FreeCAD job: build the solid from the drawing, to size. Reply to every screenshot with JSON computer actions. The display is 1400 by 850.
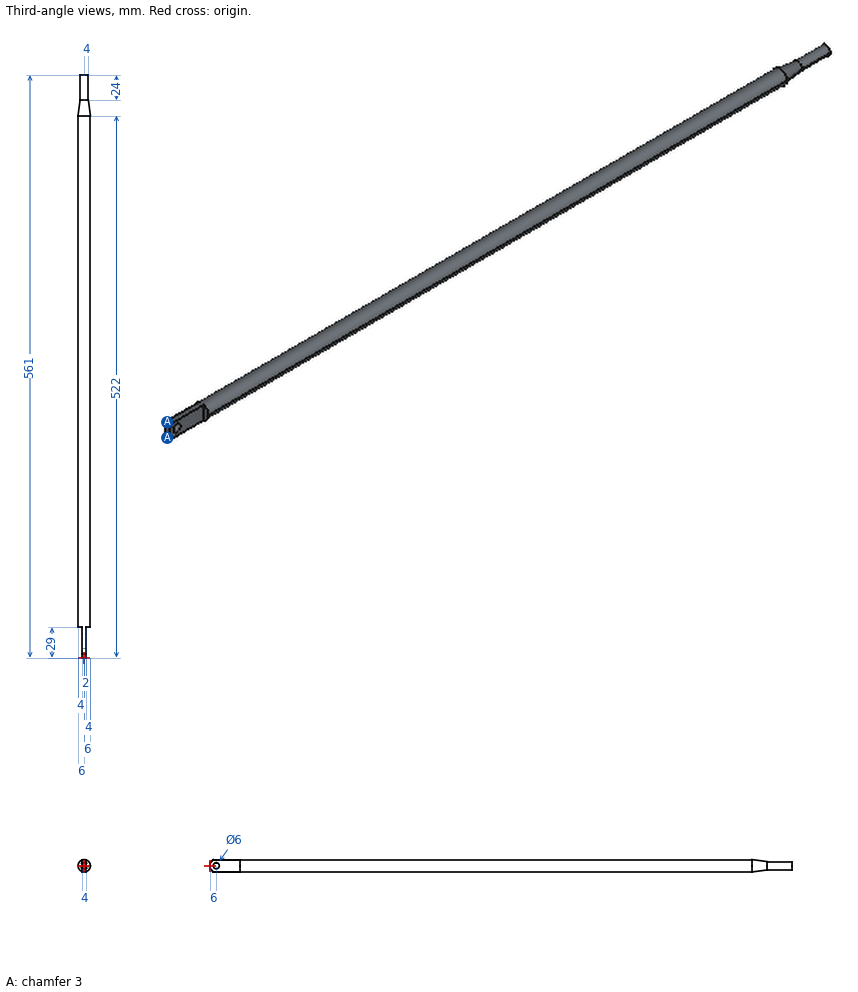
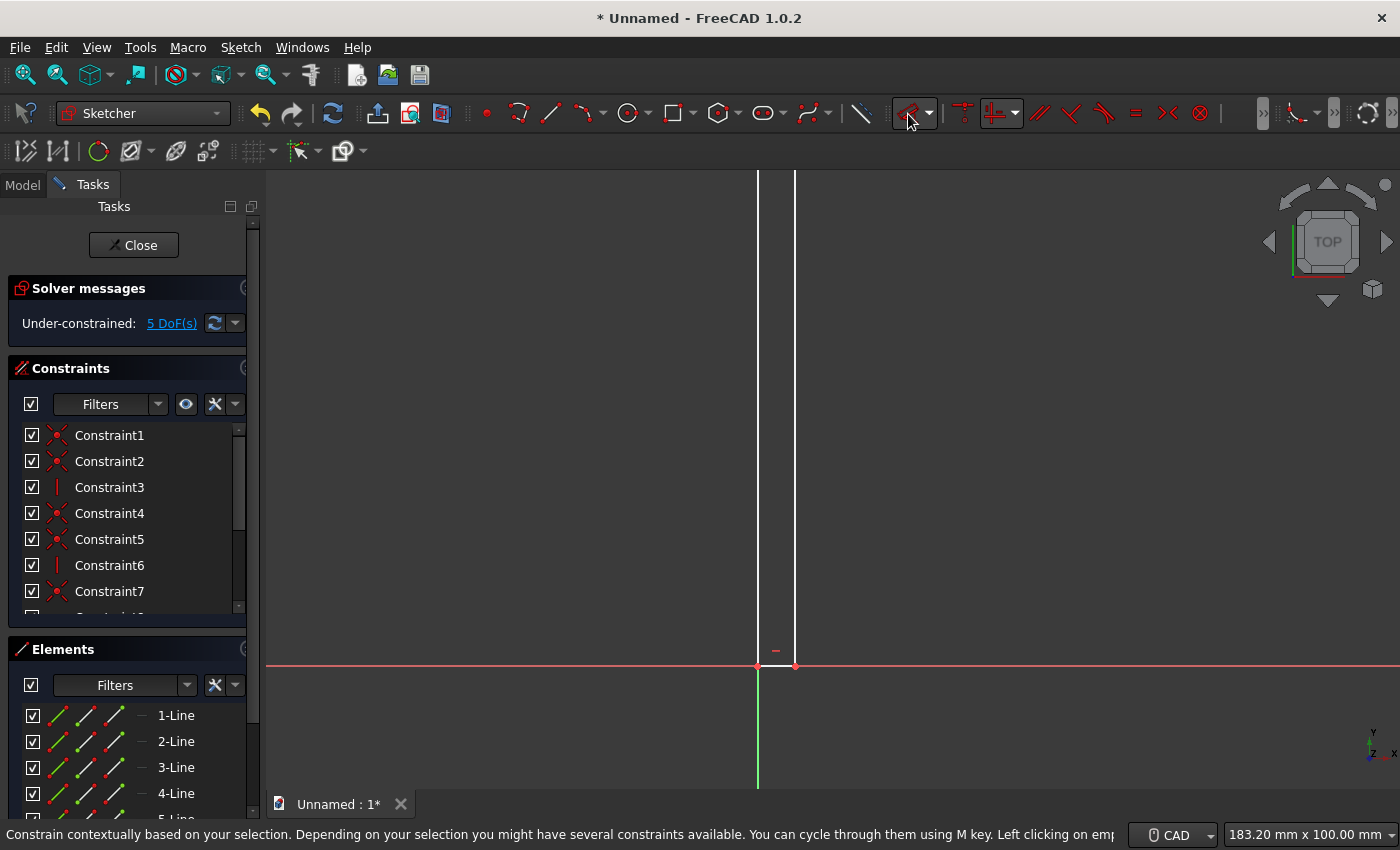
{"action": "left_click", "coordinate": [769, 666]}
{"action": "left_click", "coordinate": [777, 700]}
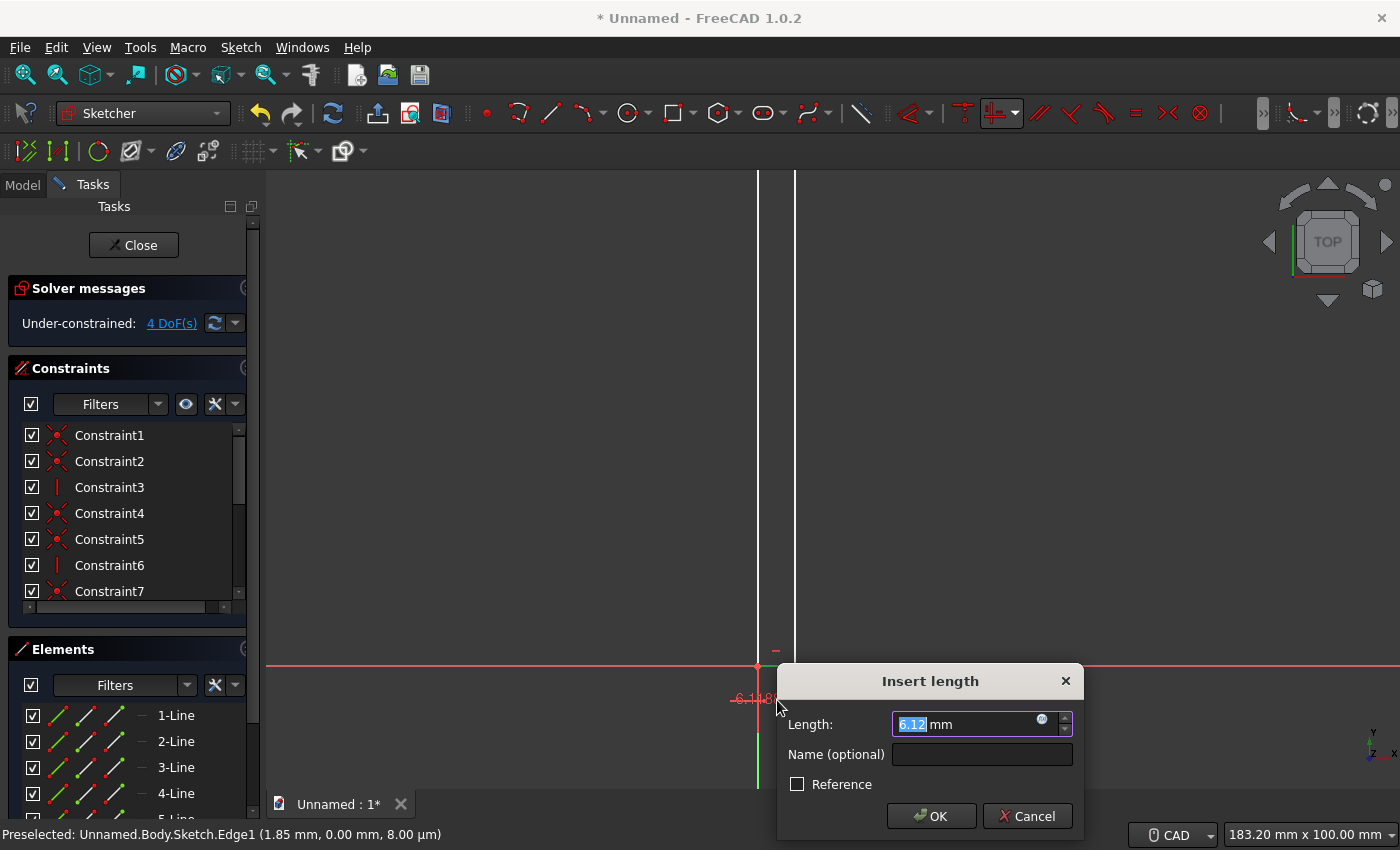
{"action": "type", "text": "6"}
{"action": "key", "text": "Return"}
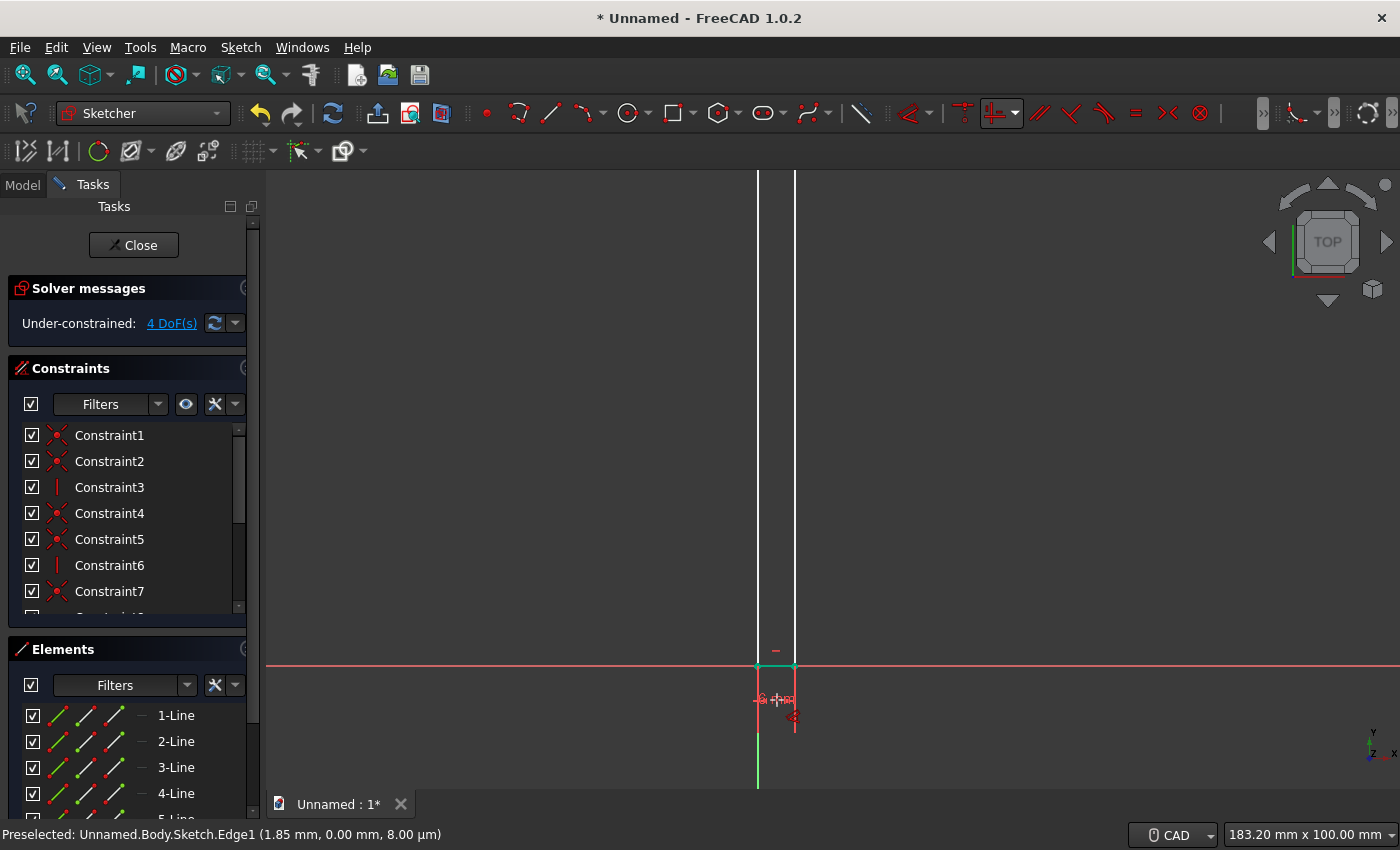
{"action": "scroll", "coordinate": [763, 673], "scroll_direction": "down", "scroll_amount": 11}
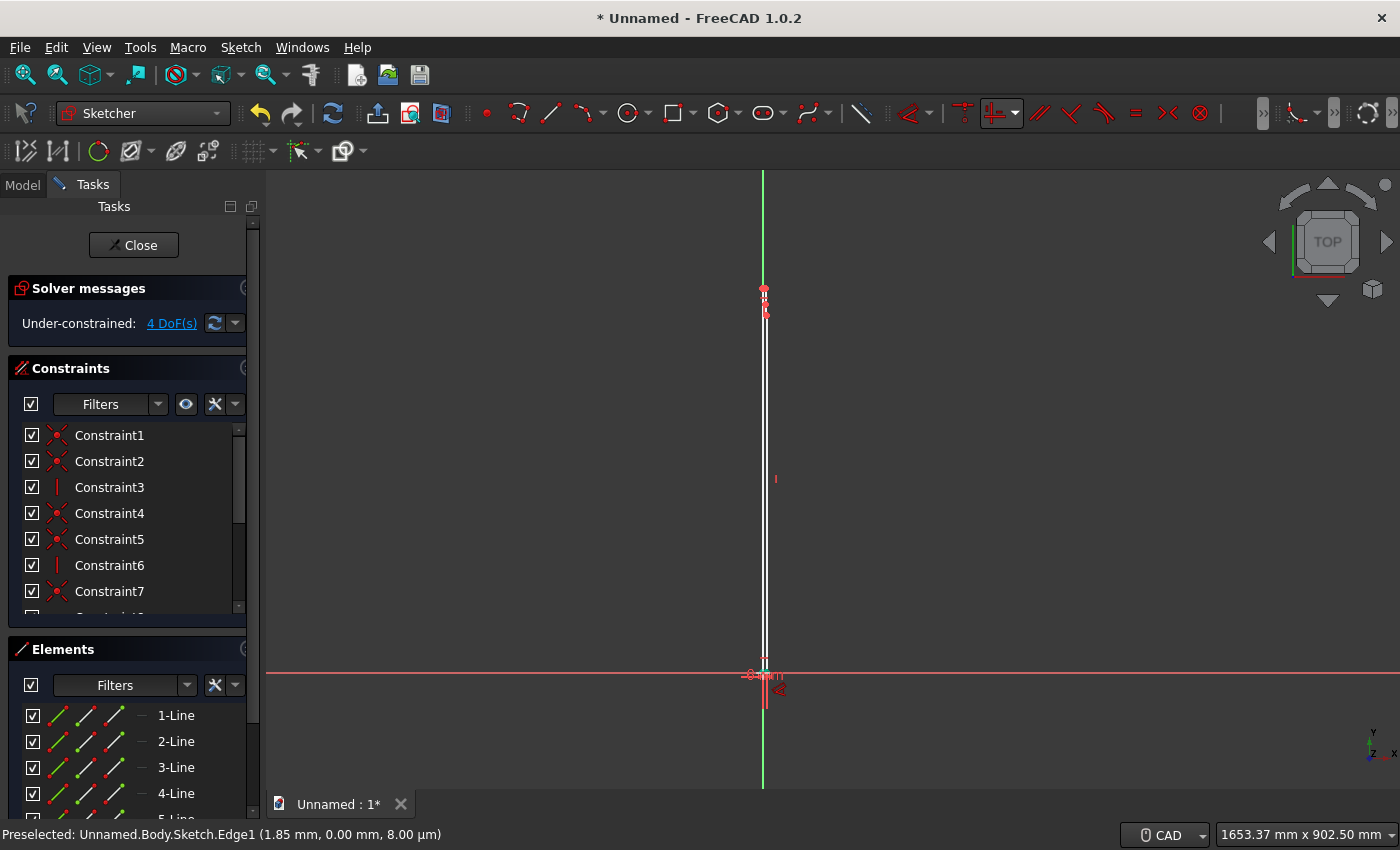
{"action": "scroll", "coordinate": [764, 288], "scroll_direction": "up", "scroll_amount": 14}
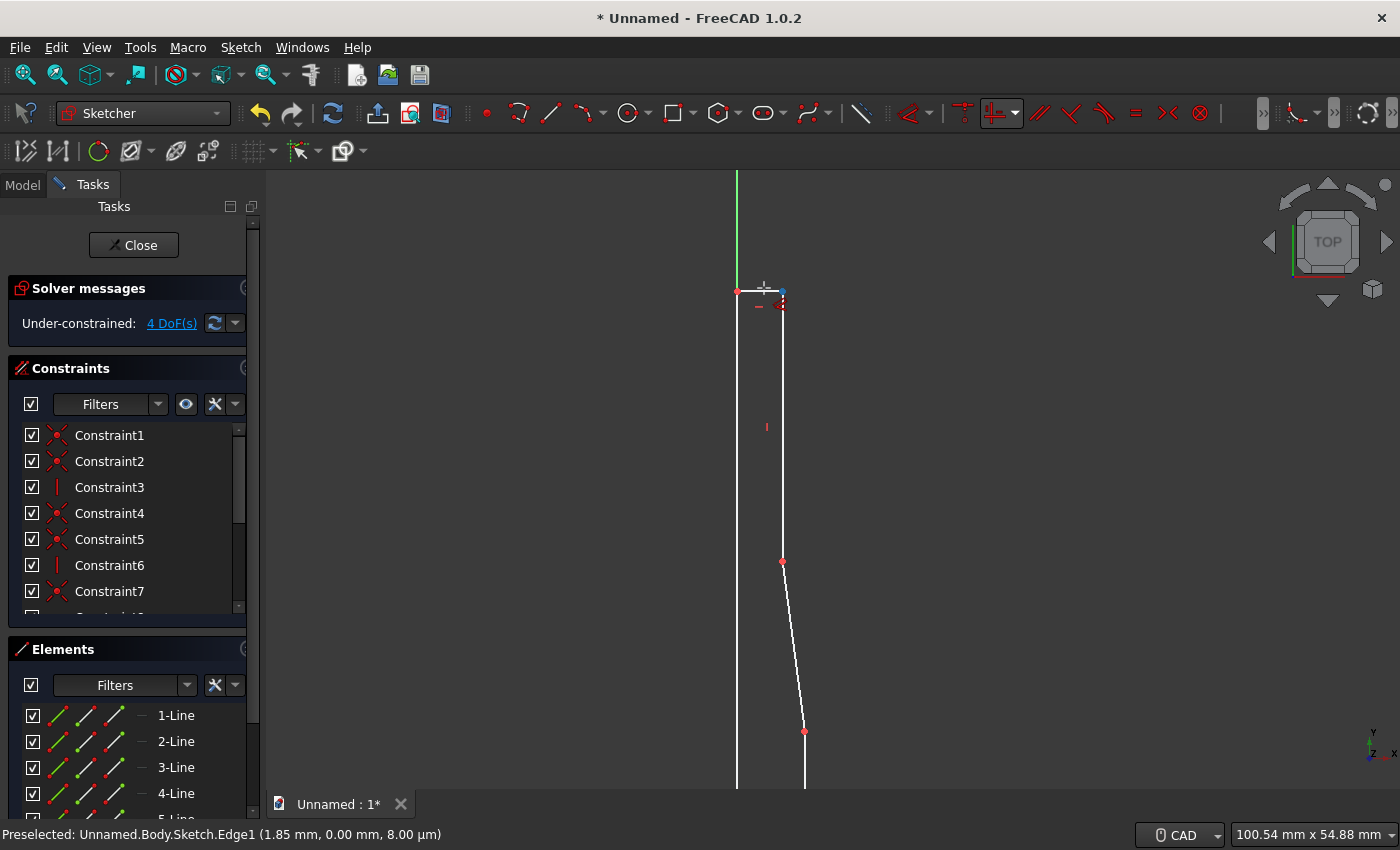
{"action": "left_click", "coordinate": [764, 291]}
{"action": "left_click", "coordinate": [760, 257]}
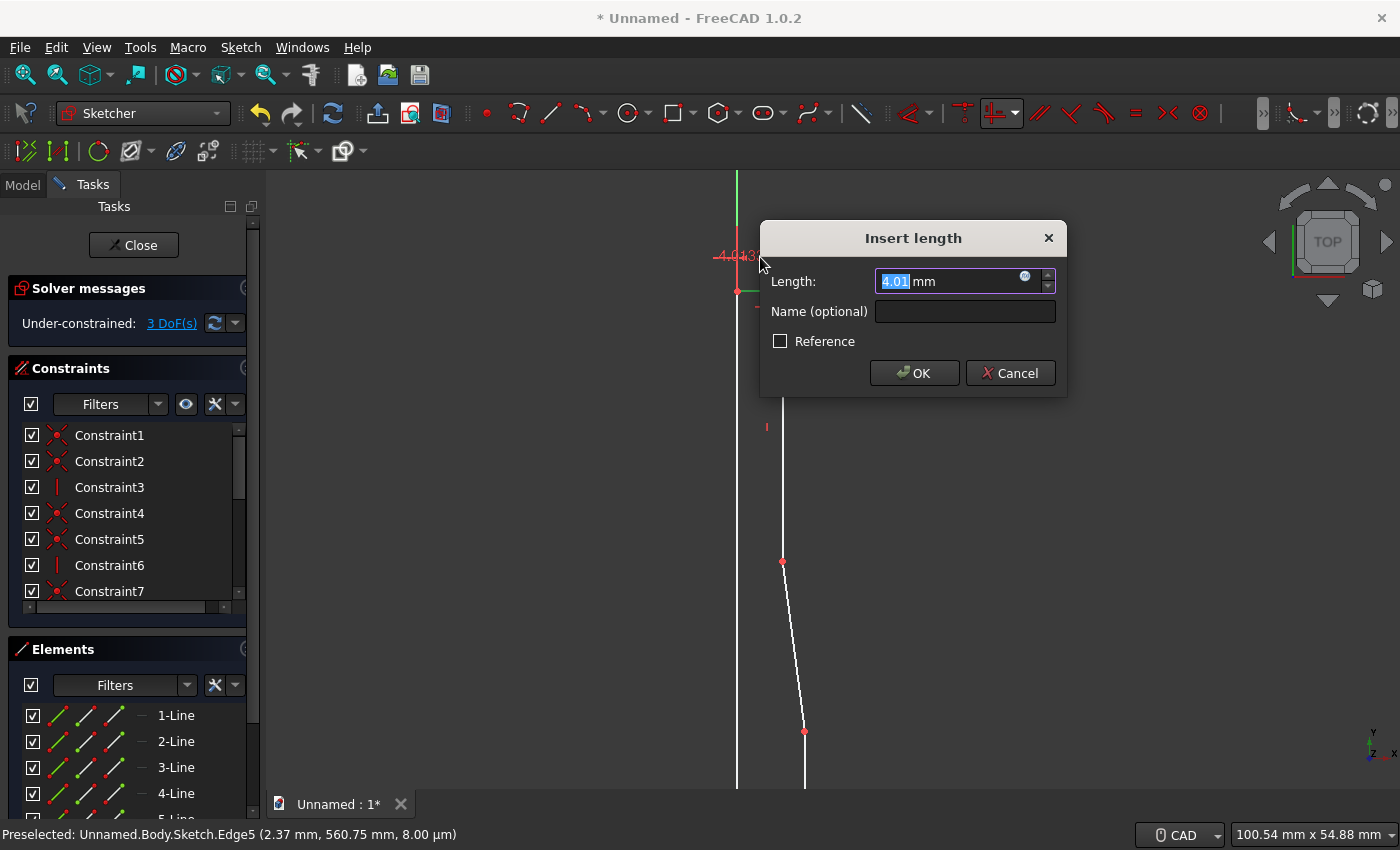
{"action": "type", "text": "4"}
{"action": "key", "text": "Return"}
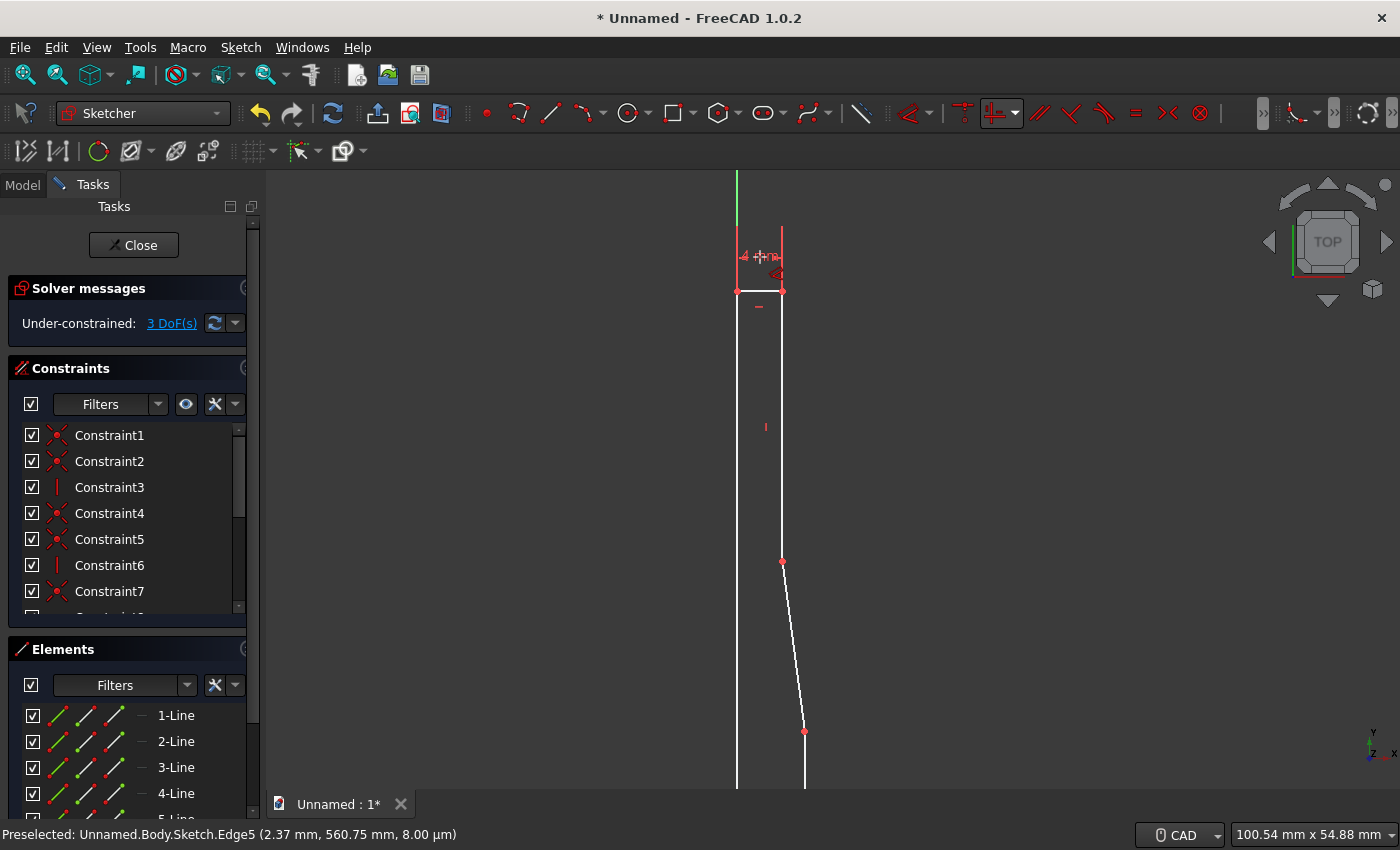
{"action": "scroll", "coordinate": [764, 287], "scroll_direction": "down", "scroll_amount": 14}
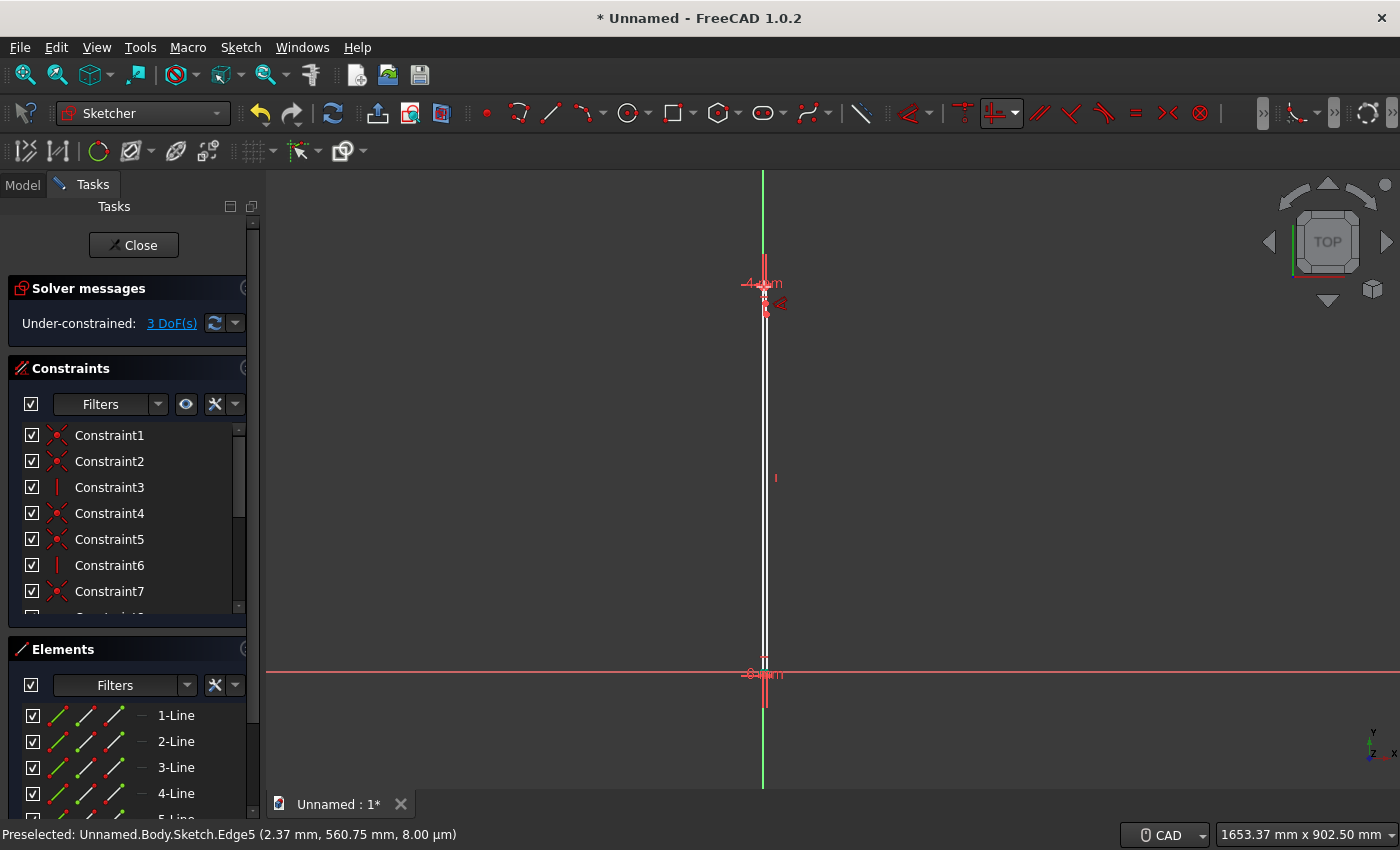
{"action": "scroll", "coordinate": [766, 299], "scroll_direction": "up", "scroll_amount": 9}